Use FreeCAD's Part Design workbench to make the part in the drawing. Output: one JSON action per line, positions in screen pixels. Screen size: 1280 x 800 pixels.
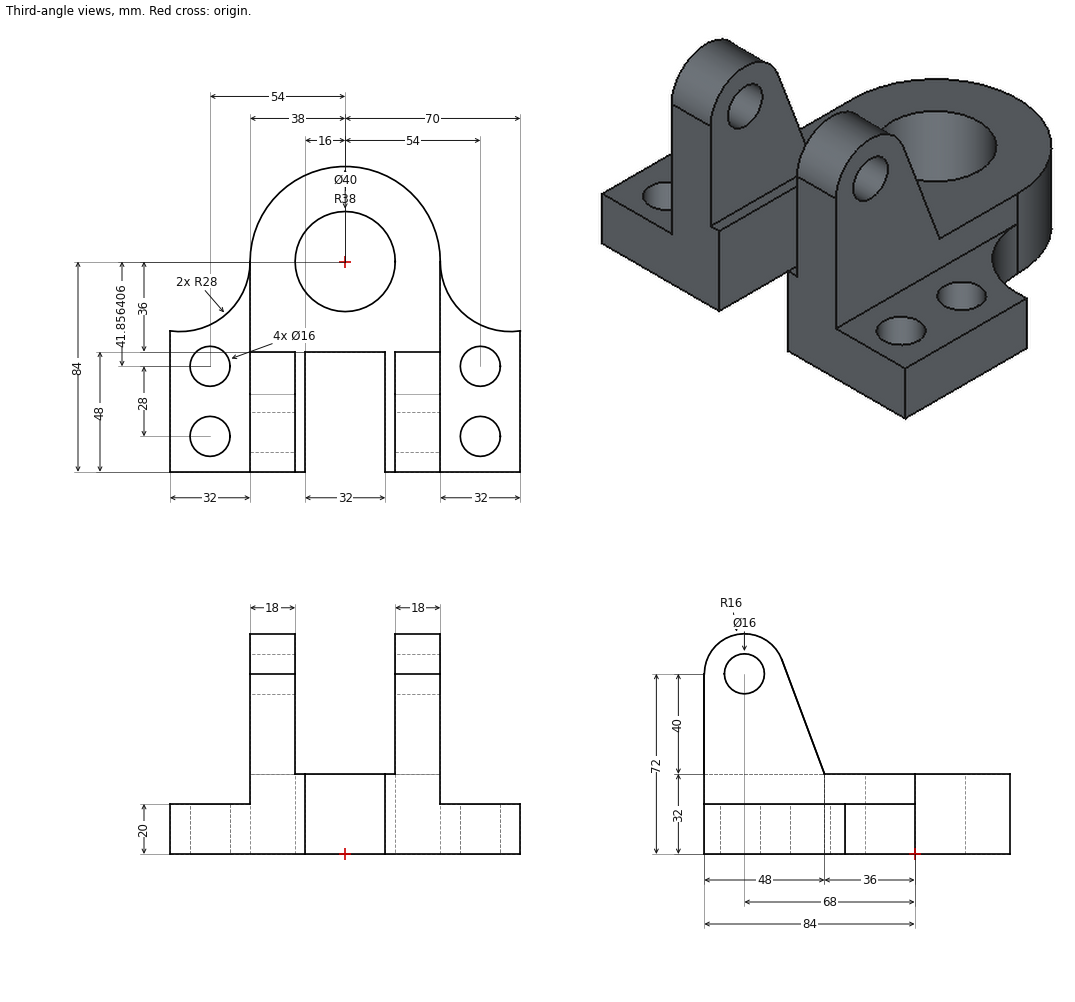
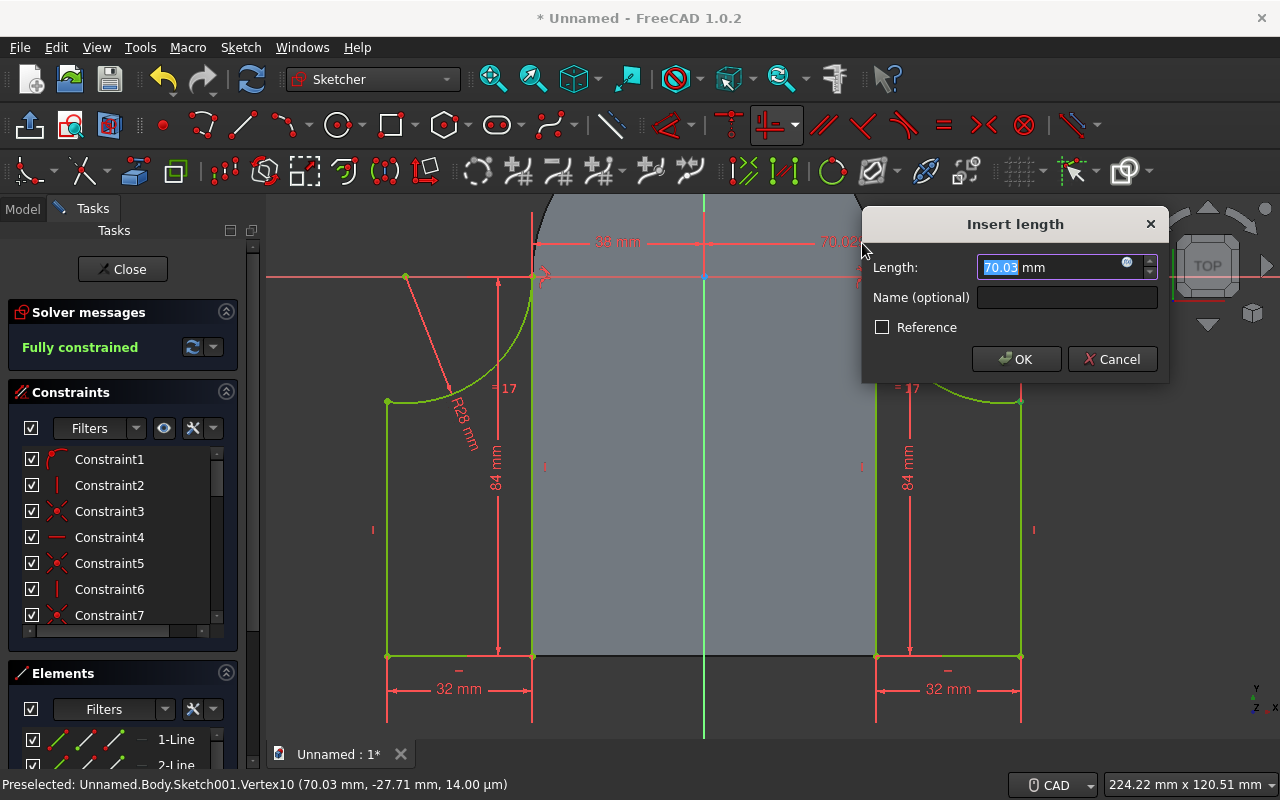
{"action": "type", "text": "70"}
{"action": "key", "text": "Return"}
{"action": "key", "text": "Escape"}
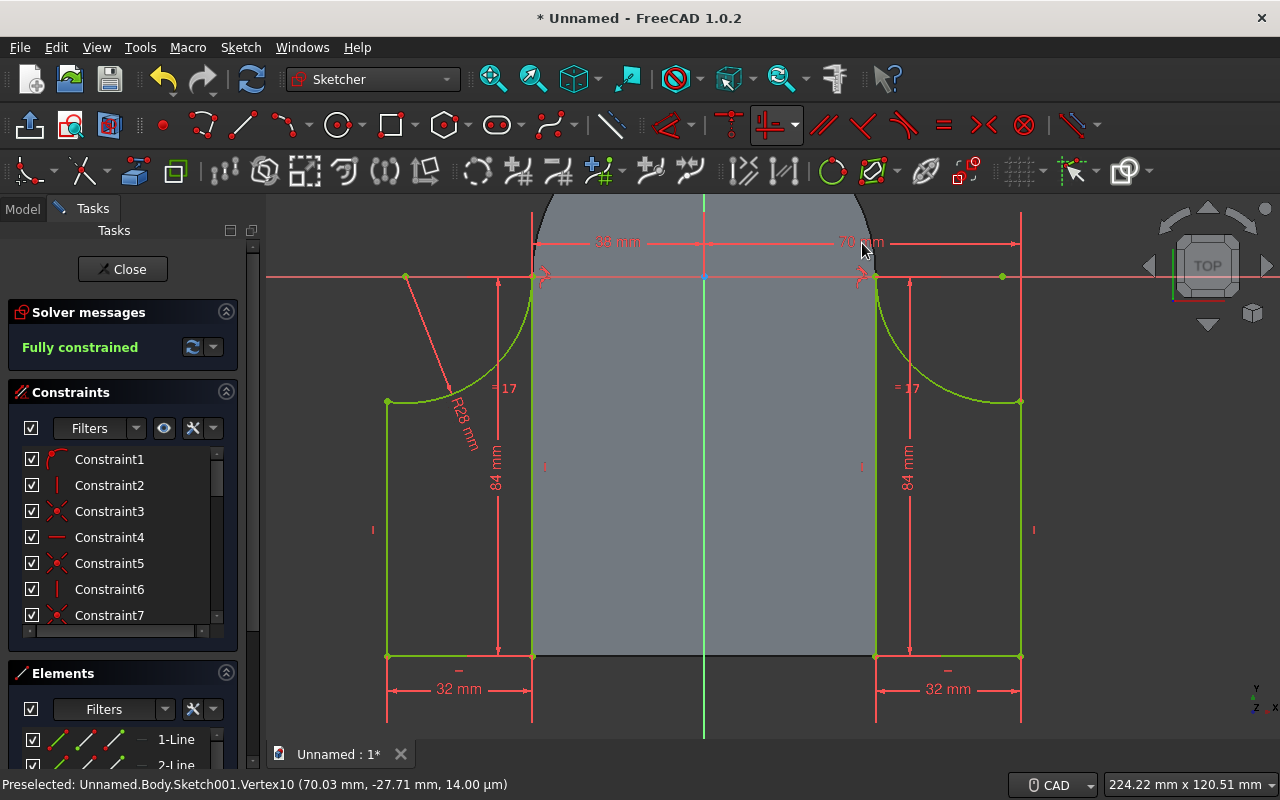
{"action": "left_click", "coordinate": [123, 269]}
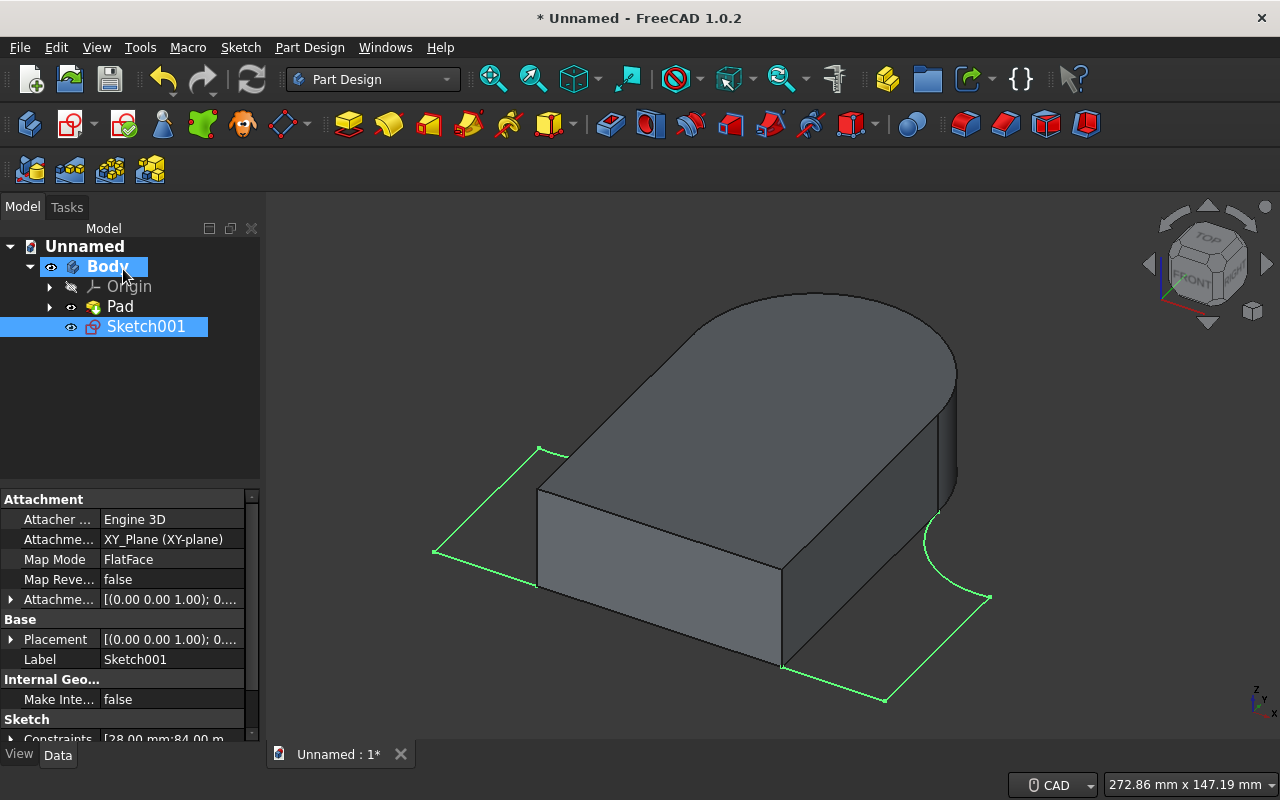
{"action": "left_click", "coordinate": [350, 124]}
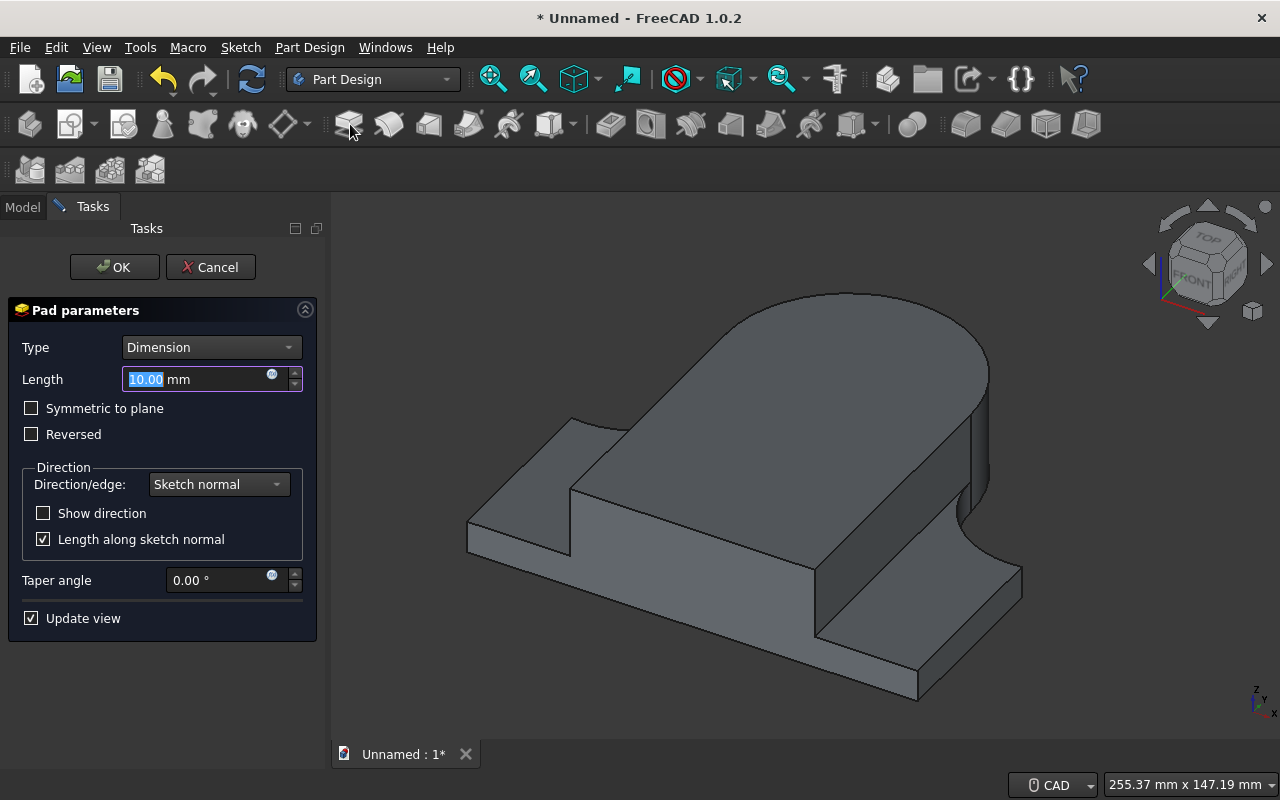
{"action": "type", "text": "20"}
{"action": "key", "text": "Tab"}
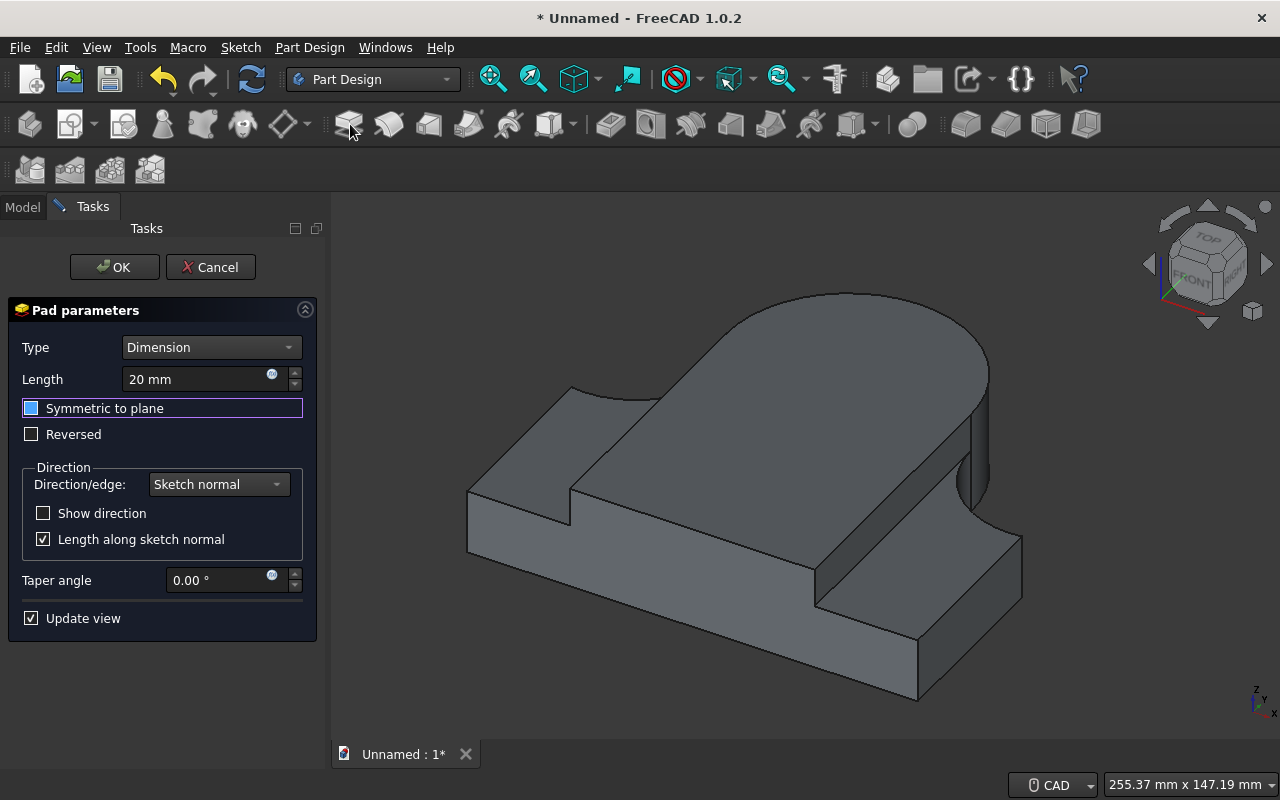
{"action": "left_click", "coordinate": [115, 267]}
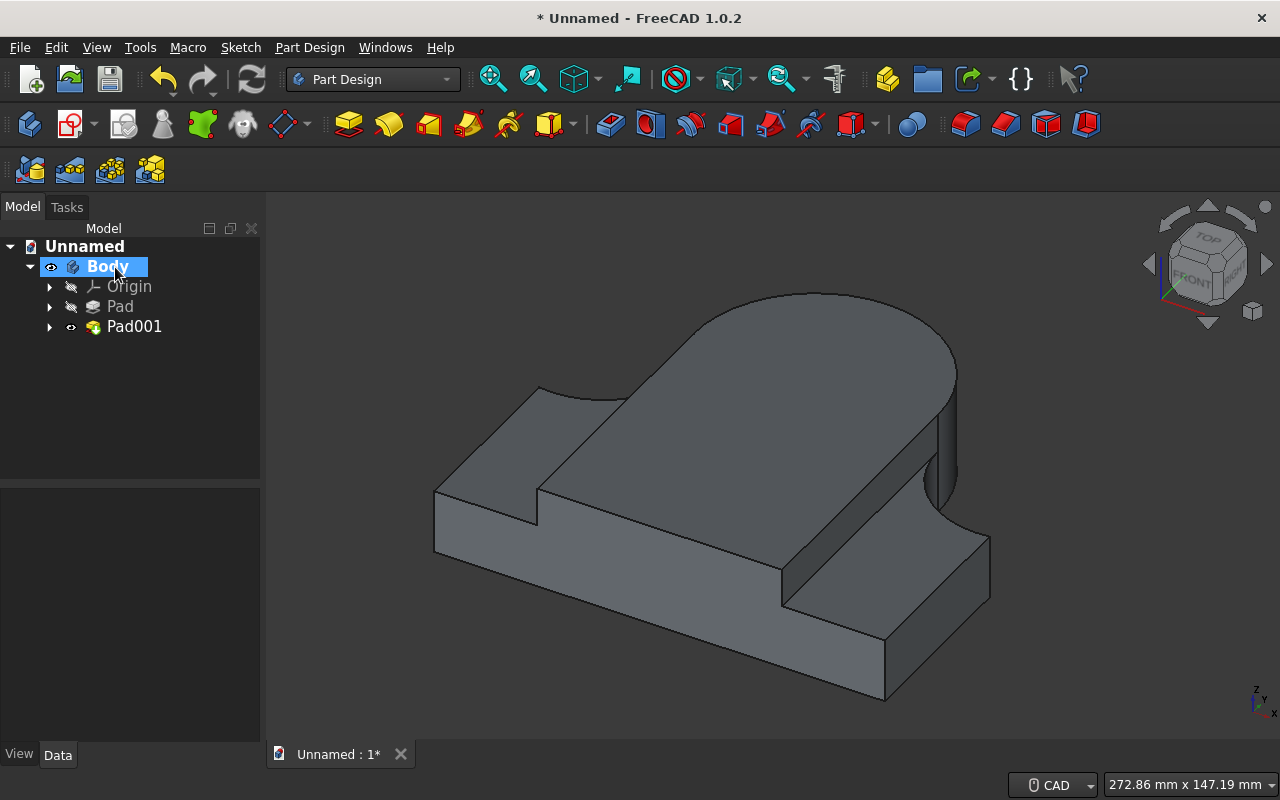
{"action": "key", "text": "6"}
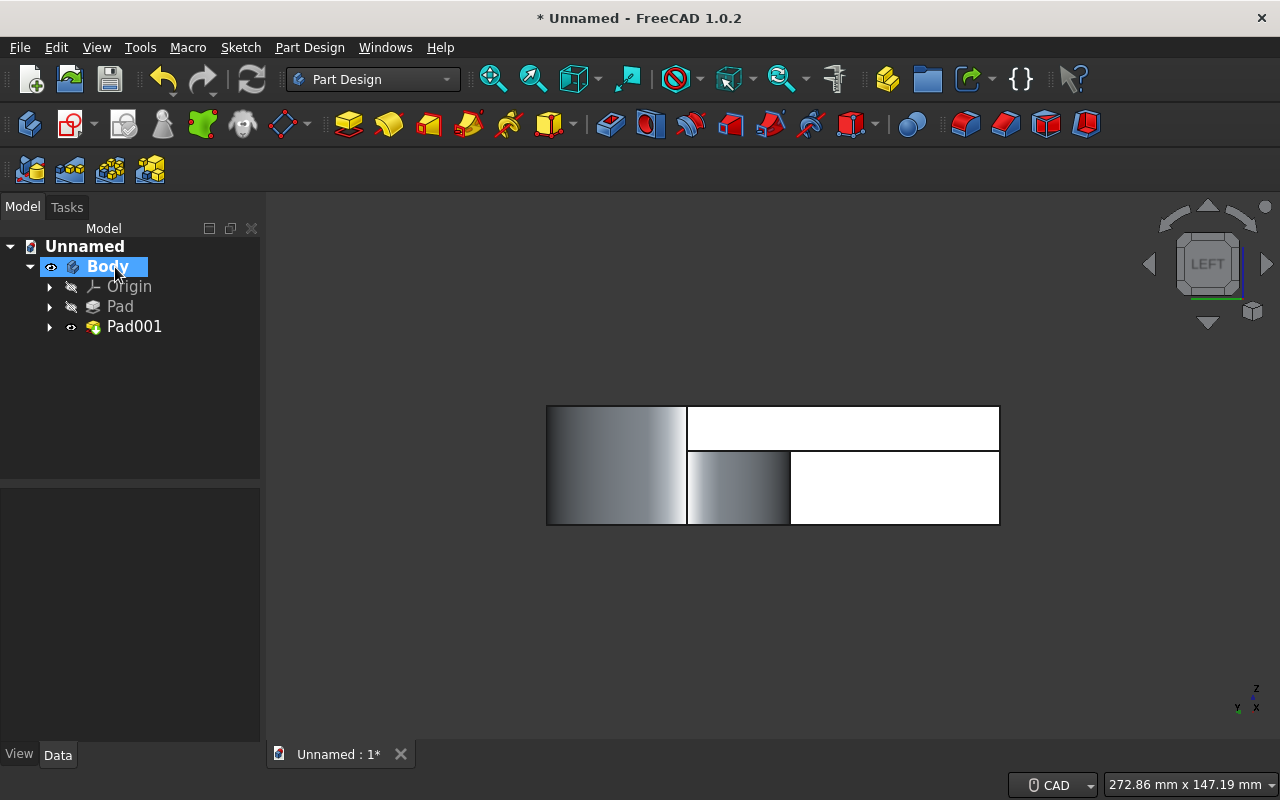
{"action": "left_click", "coordinate": [494, 80]}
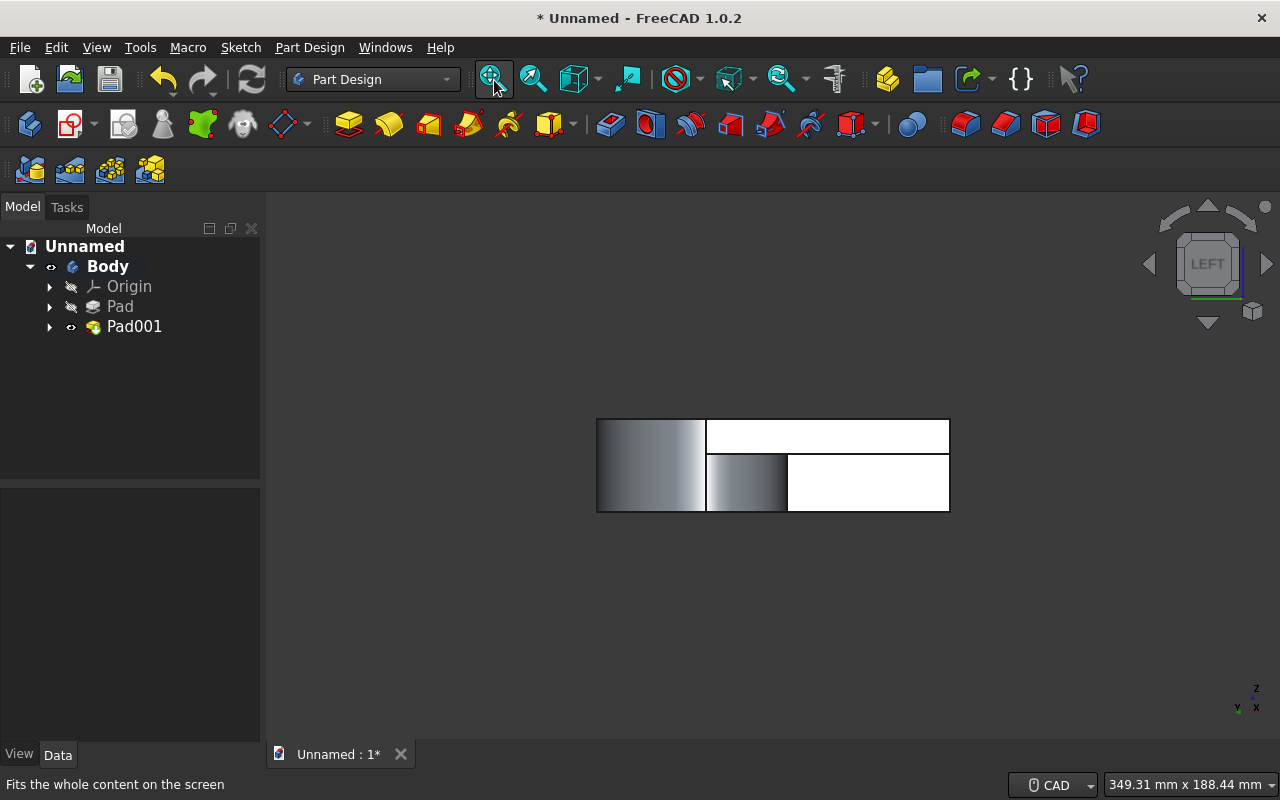
{"action": "left_click", "coordinate": [724, 435]}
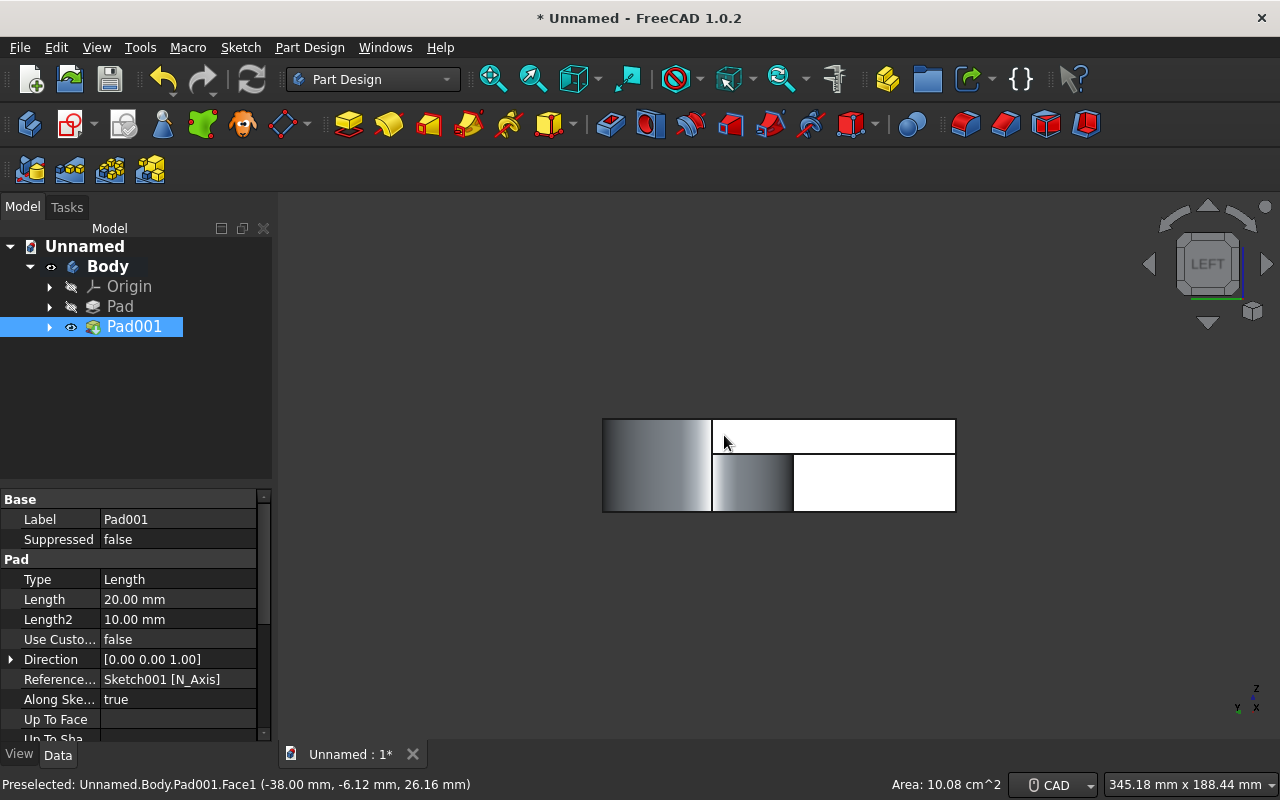
{"action": "left_click", "coordinate": [70, 124]}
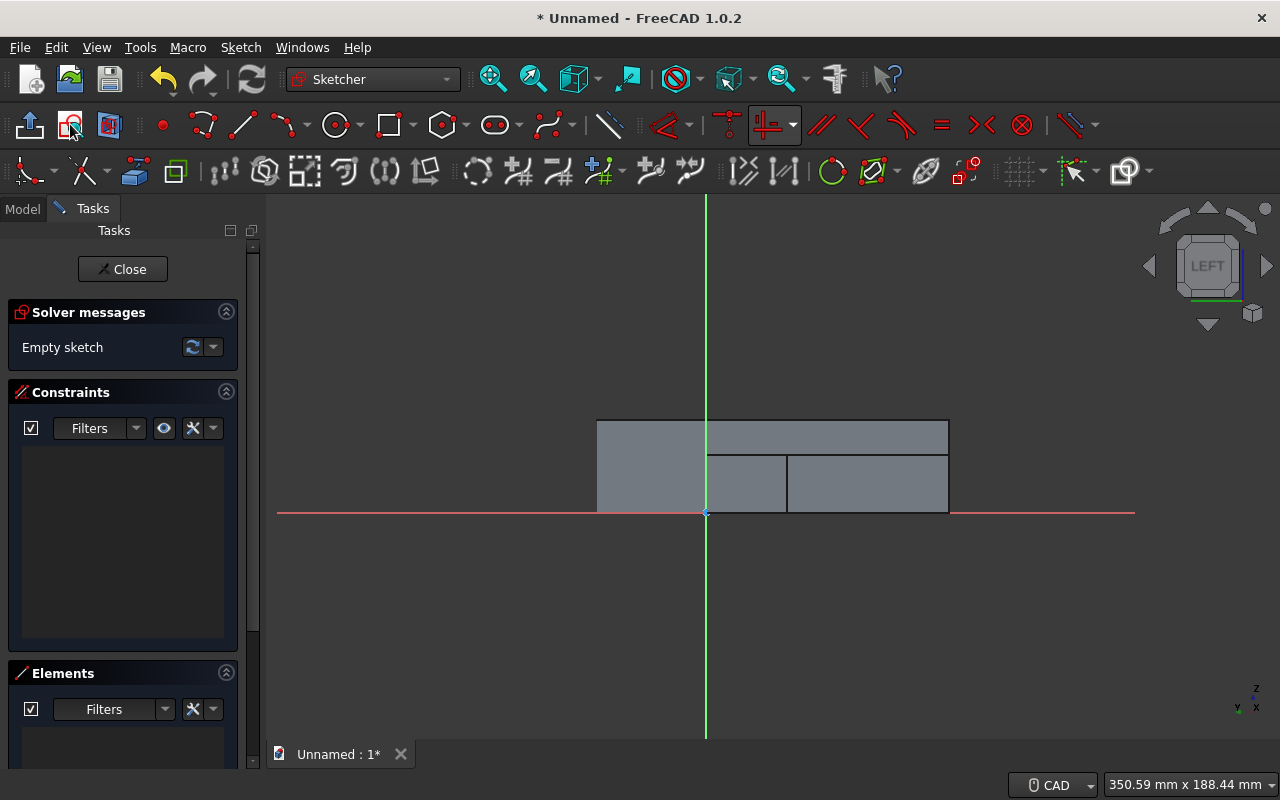
{"action": "left_click", "coordinate": [110, 126]}